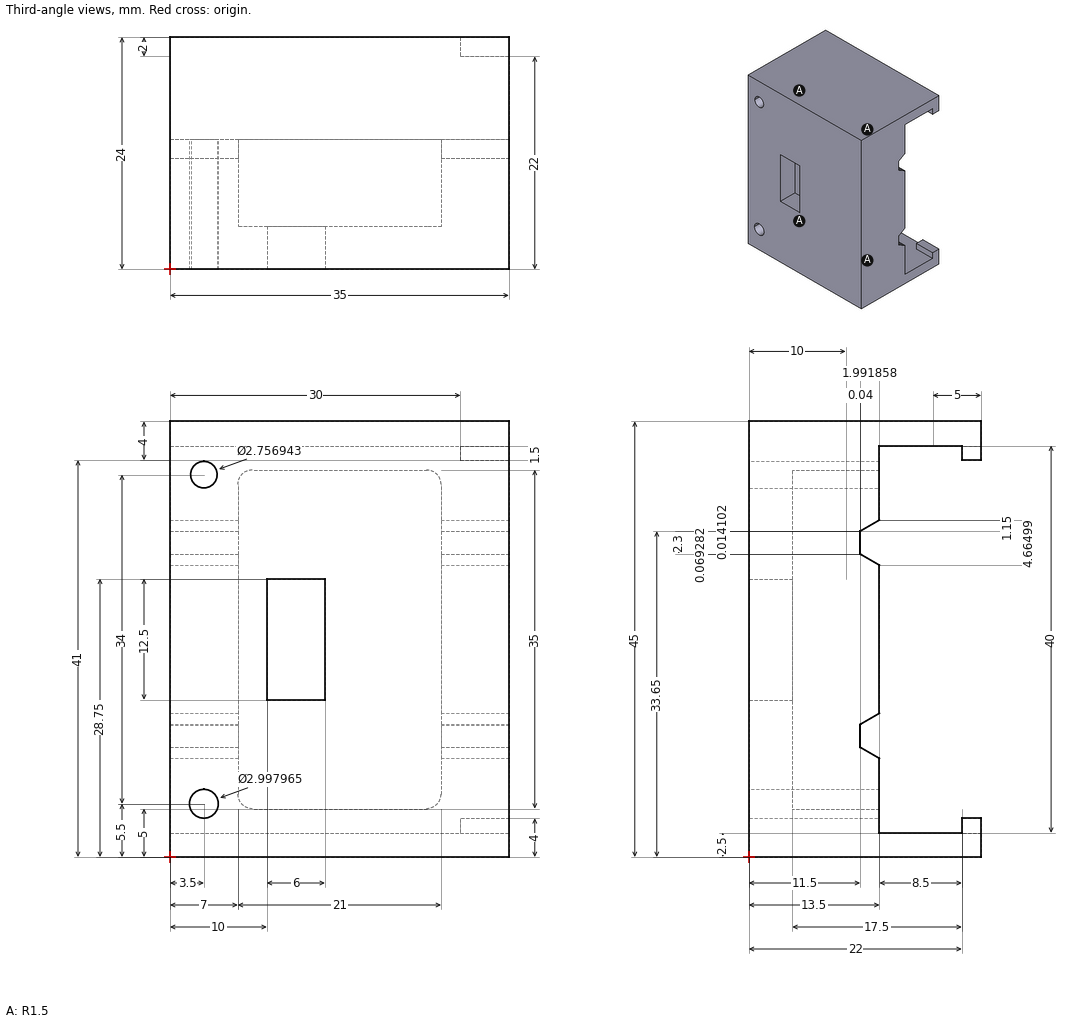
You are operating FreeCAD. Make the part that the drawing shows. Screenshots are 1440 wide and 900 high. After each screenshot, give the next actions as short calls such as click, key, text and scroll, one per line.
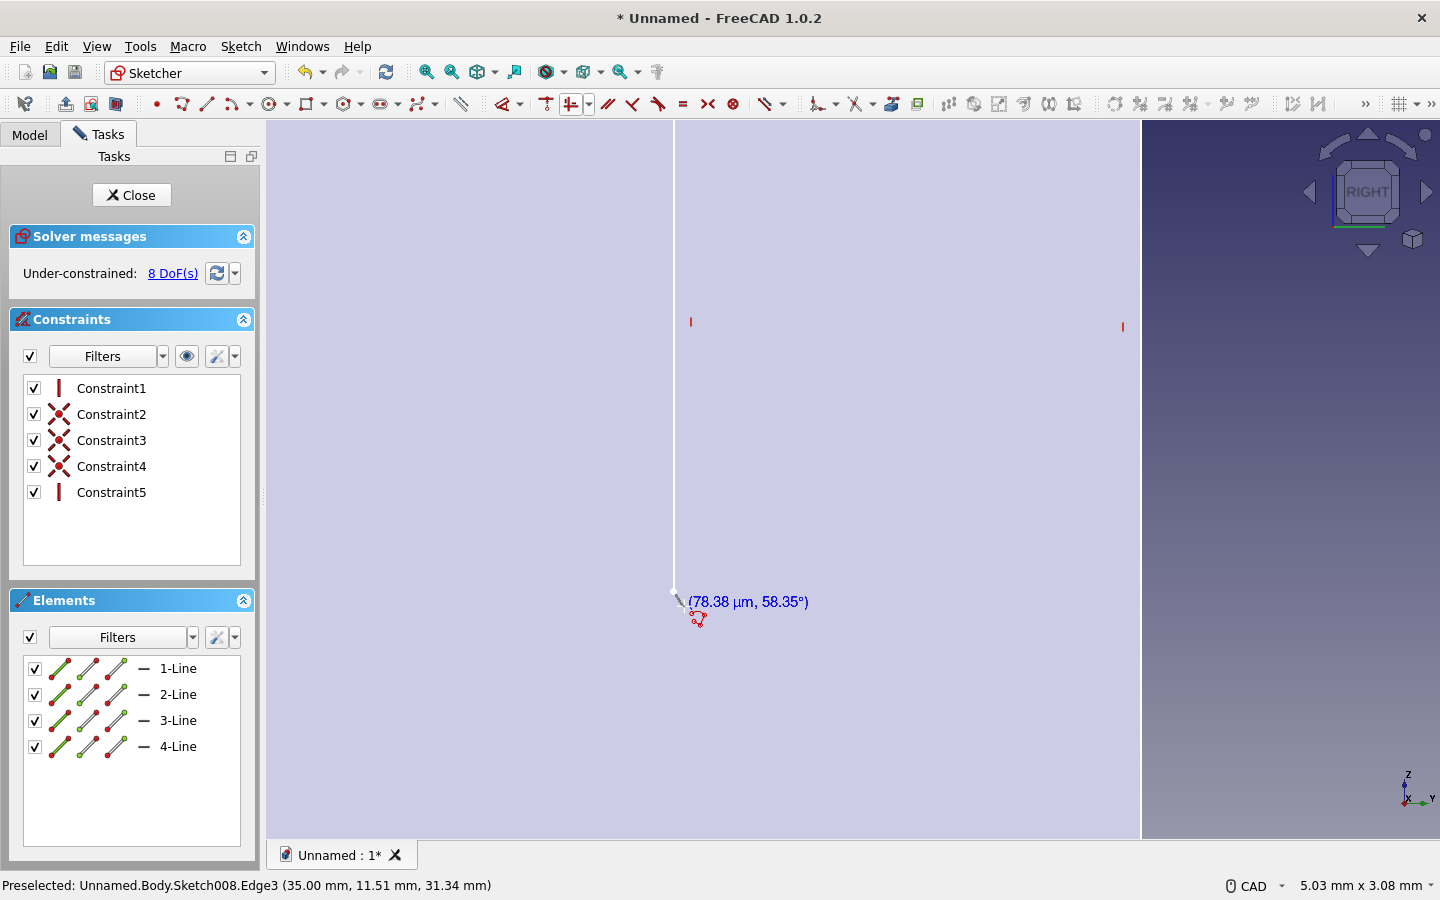
click(683, 605)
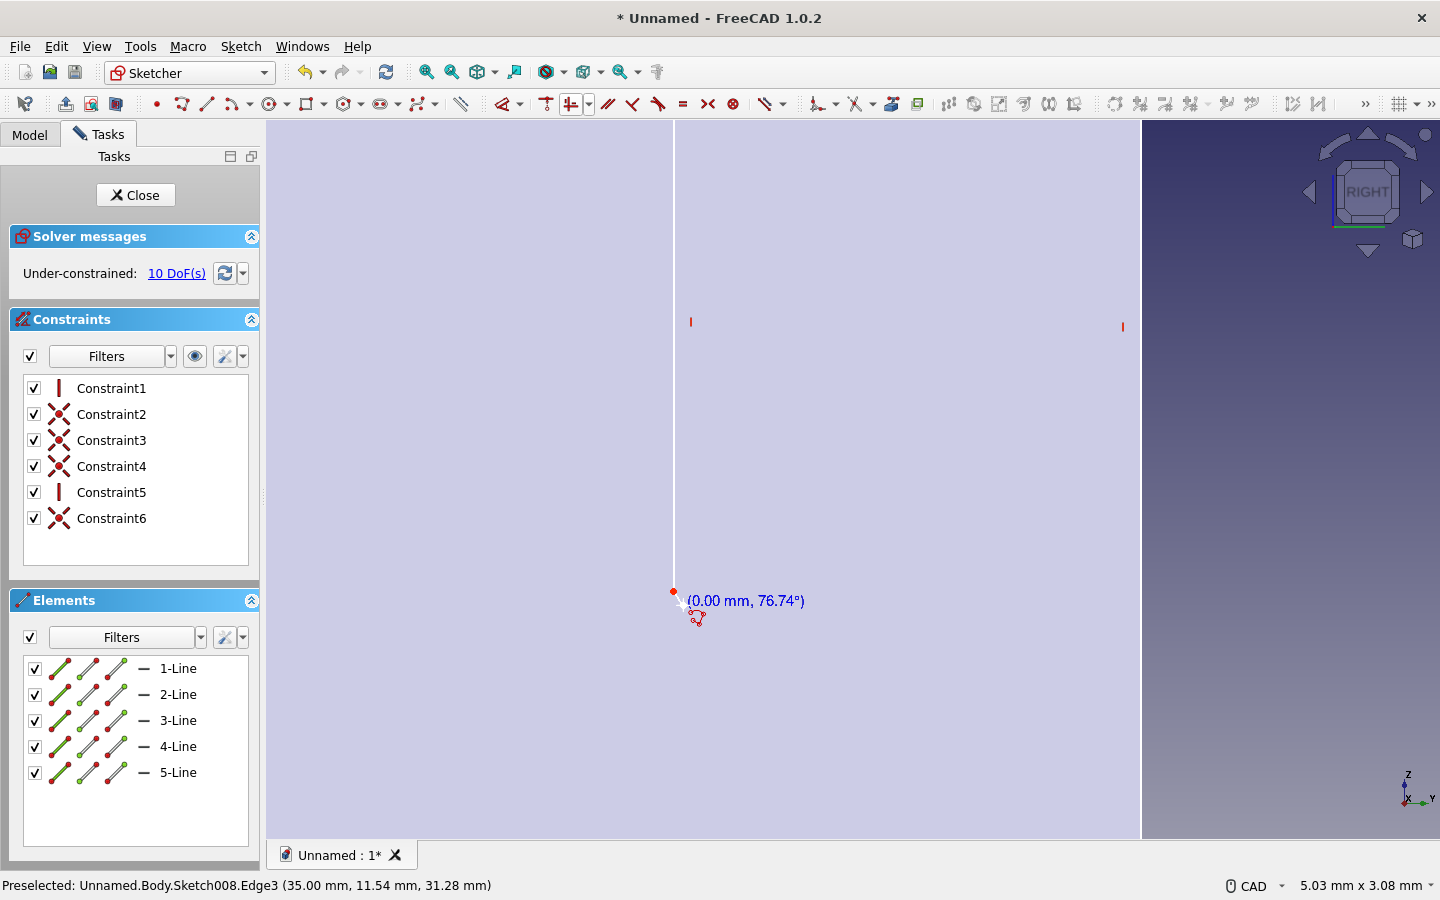
scroll(684, 606, down, 4)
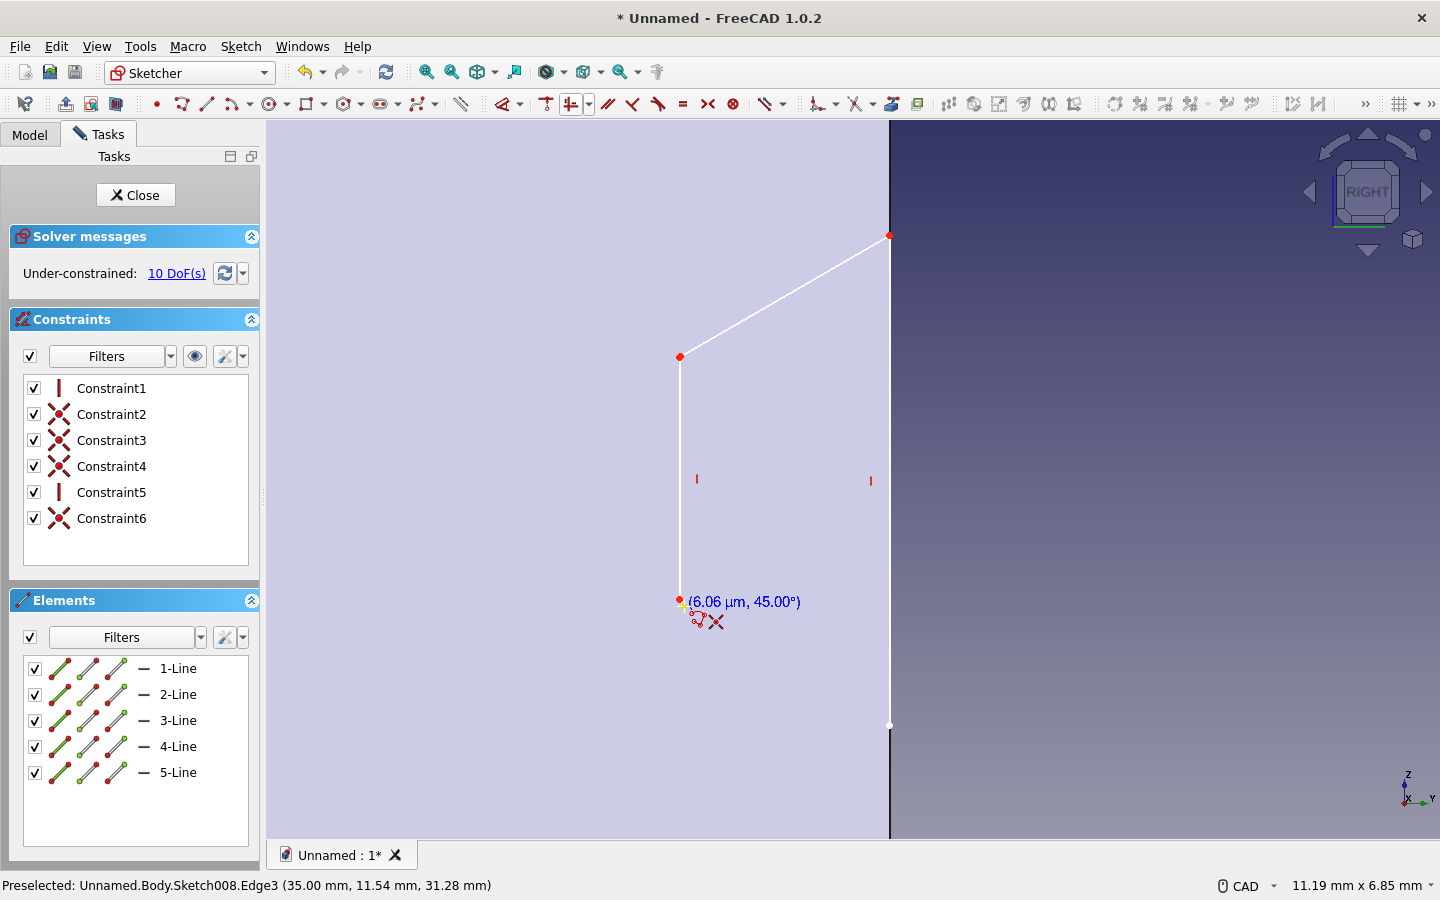
click(890, 726)
key(Escape)
key(Escape)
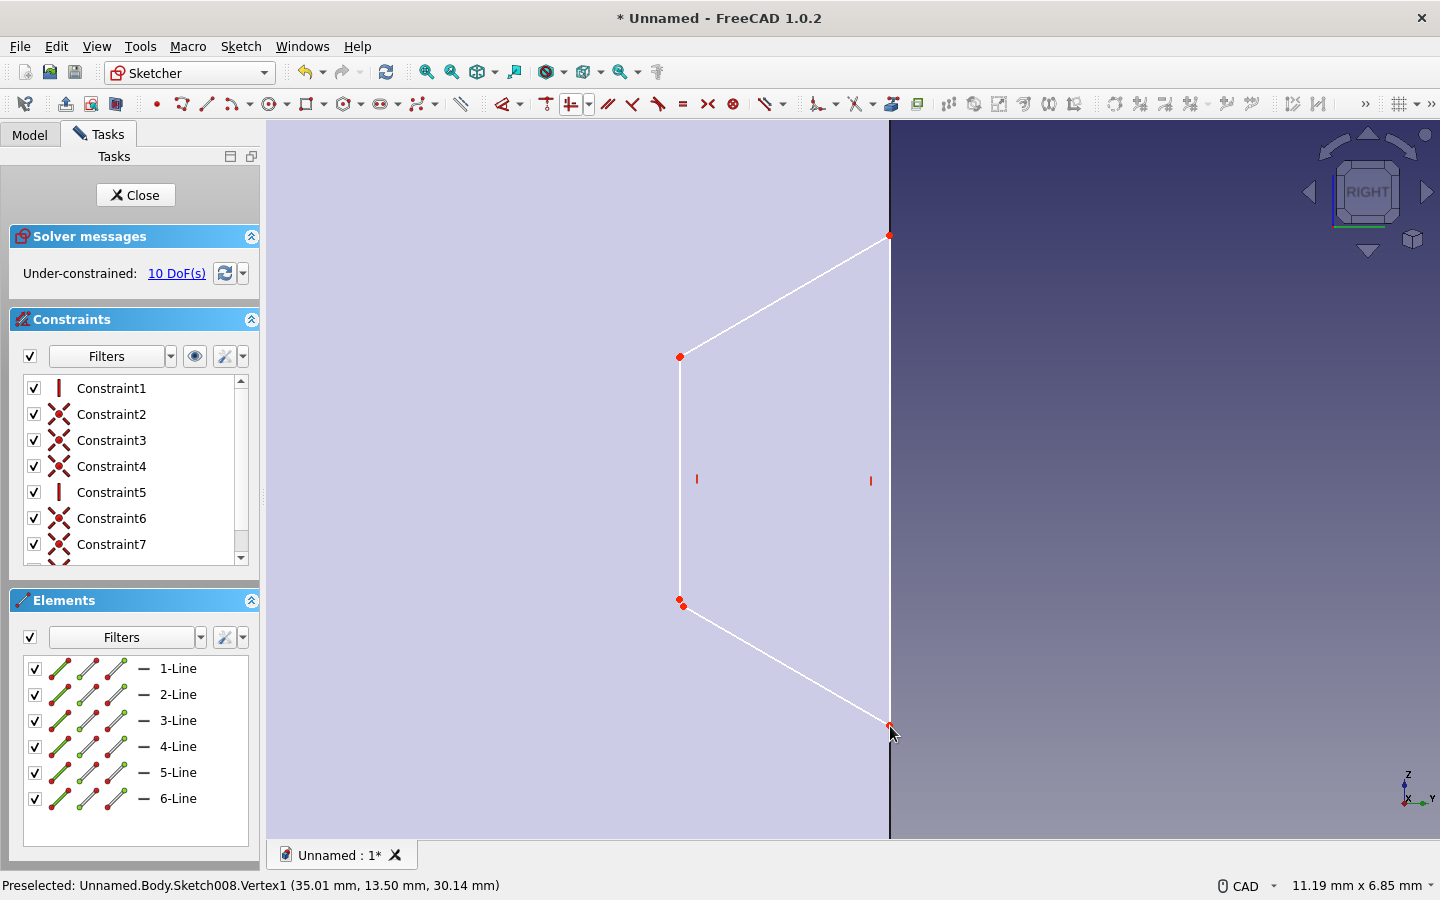
click(502, 104)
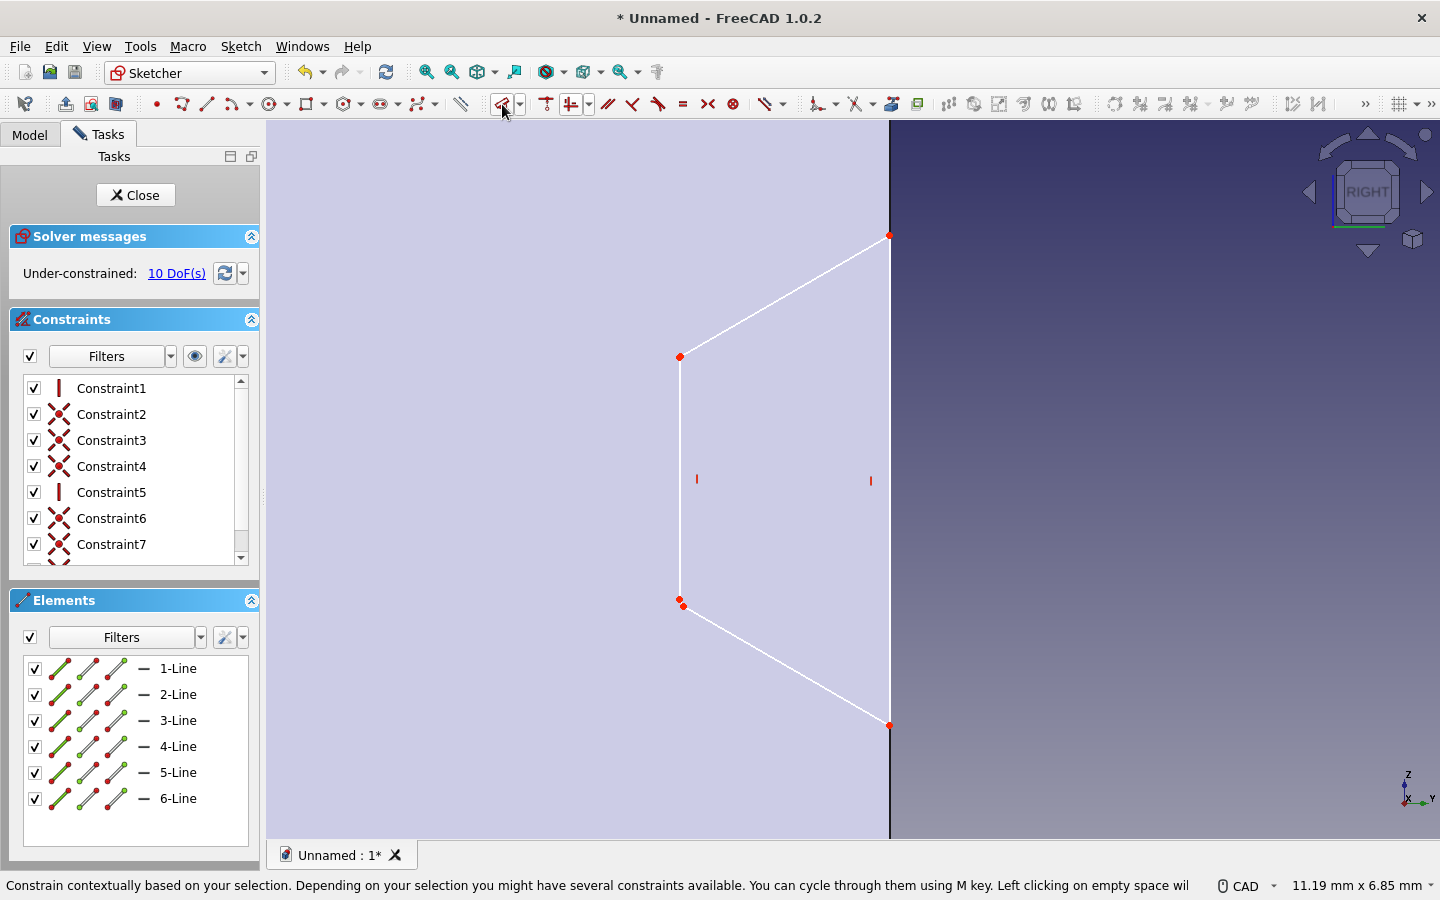
click(680, 430)
click(646, 479)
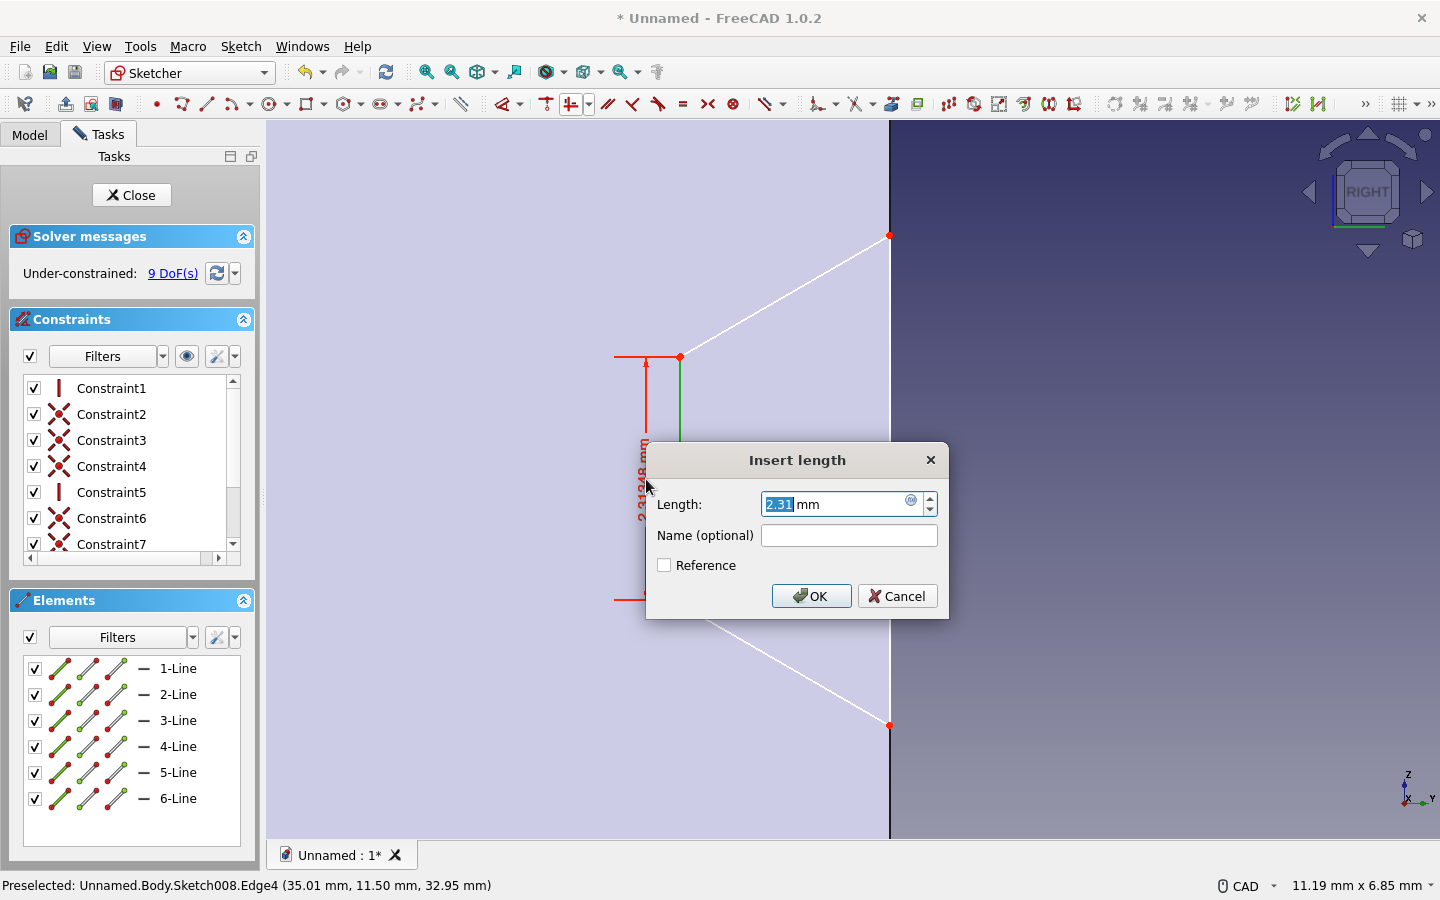
text(2.3)
key(Return)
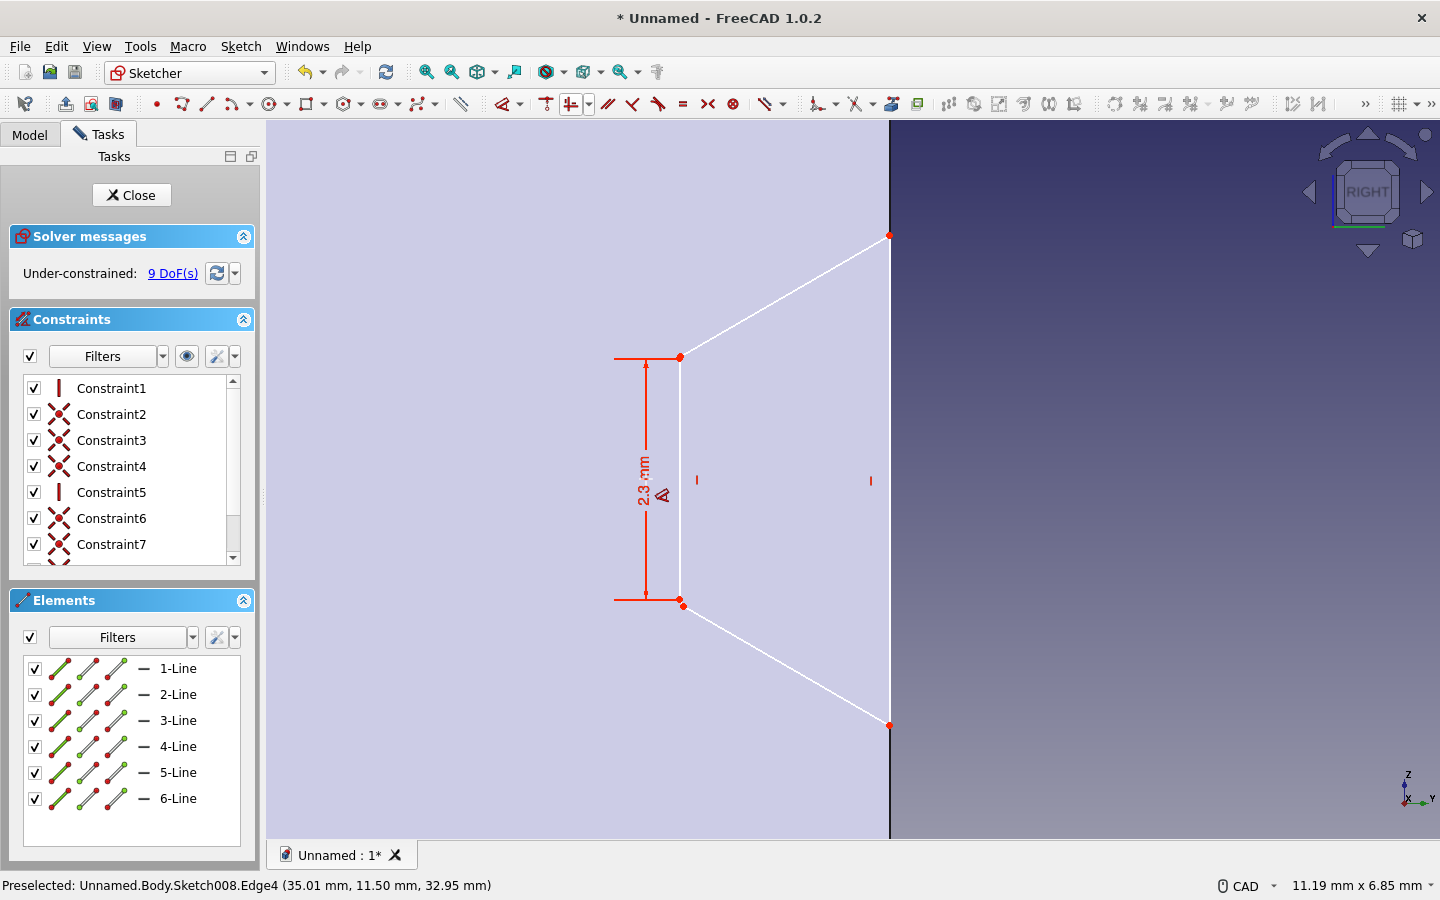
click(890, 726)
click(592, 692)